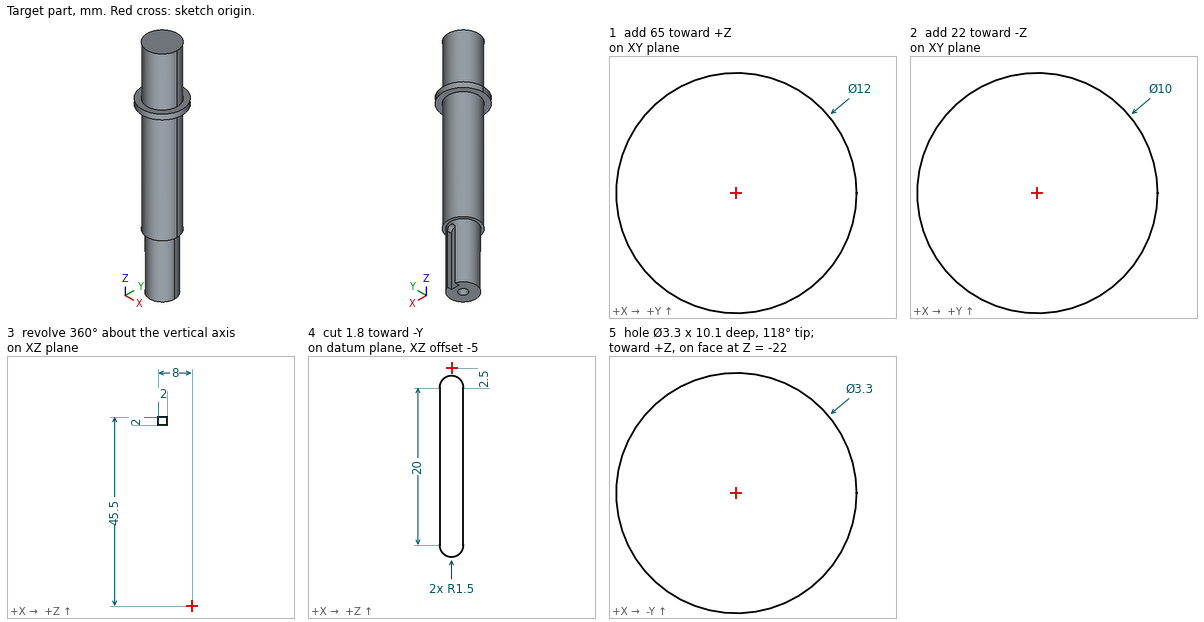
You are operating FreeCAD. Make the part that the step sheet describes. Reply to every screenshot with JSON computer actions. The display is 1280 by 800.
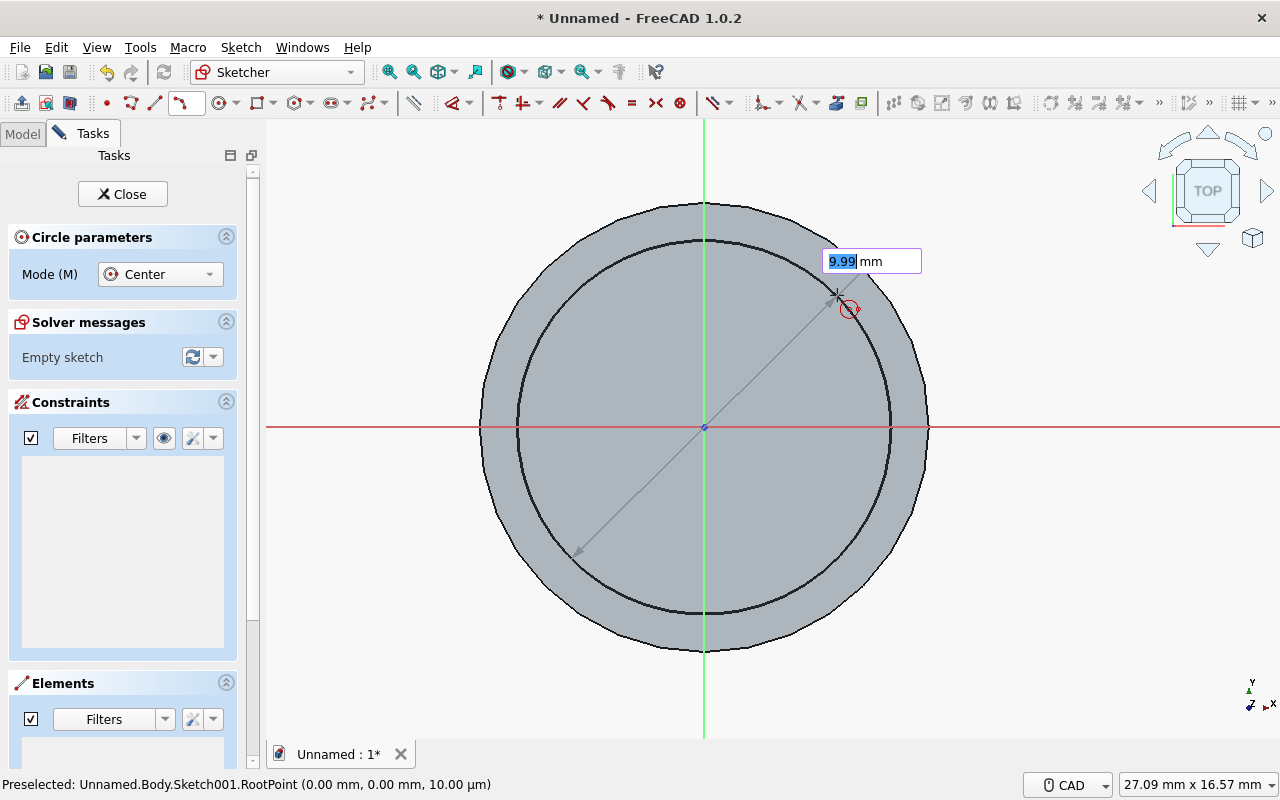
{"action": "type", "text": "10"}
{"action": "key", "text": "Return"}
{"action": "key", "text": "Escape"}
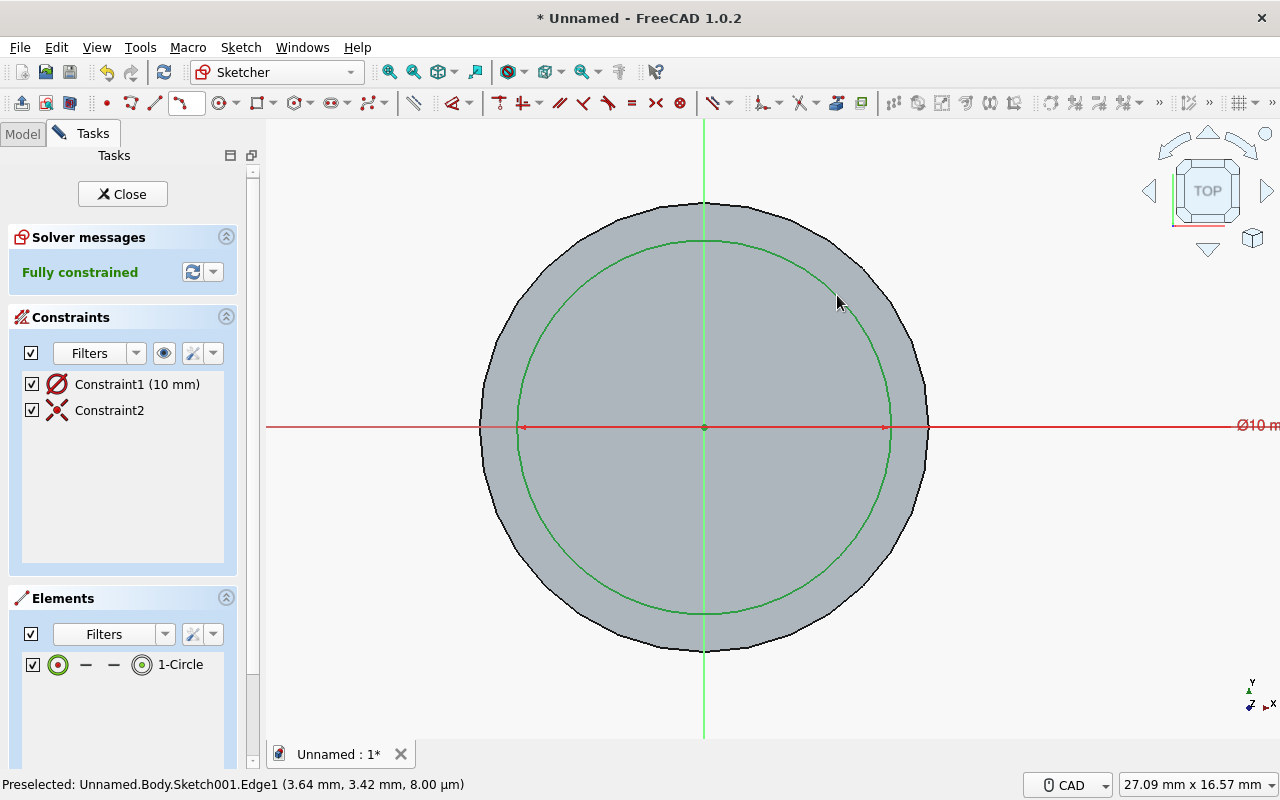
{"action": "left_click", "coordinate": [123, 194]}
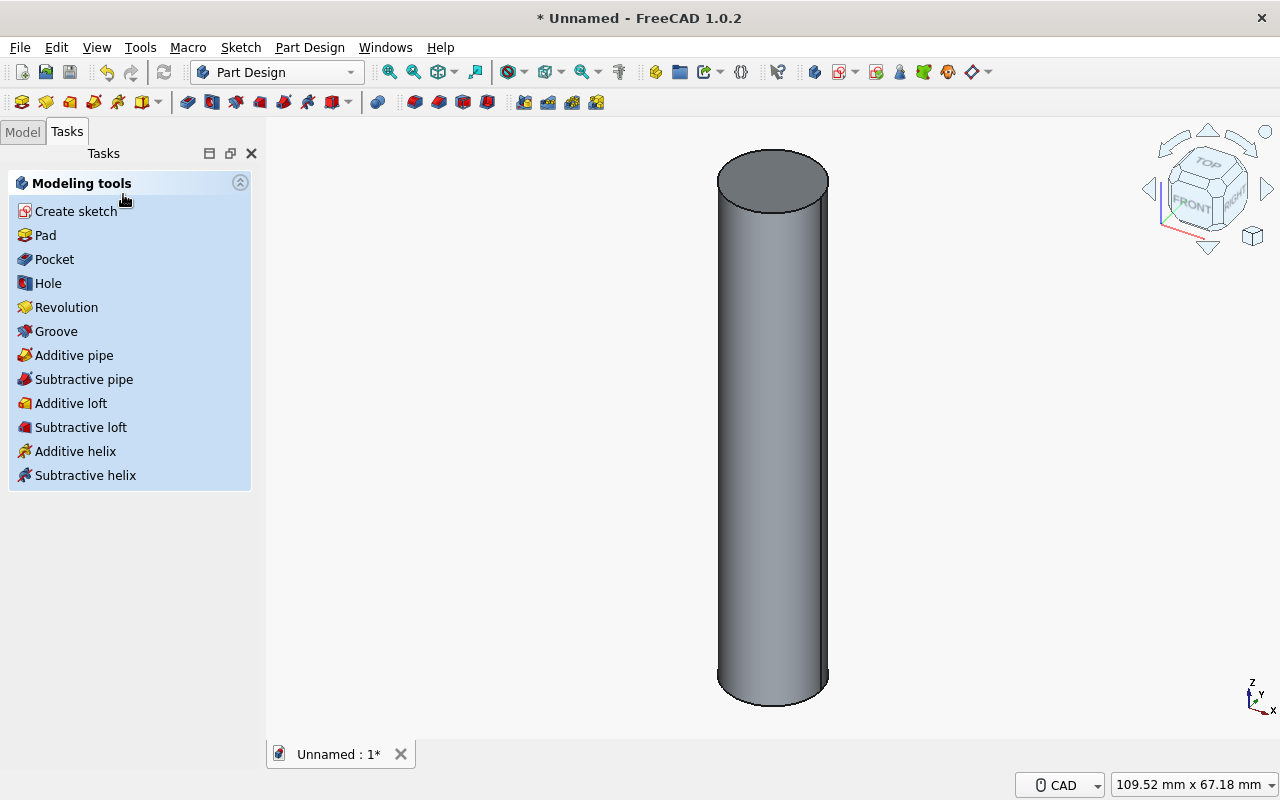
{"action": "left_click", "coordinate": [22, 102]}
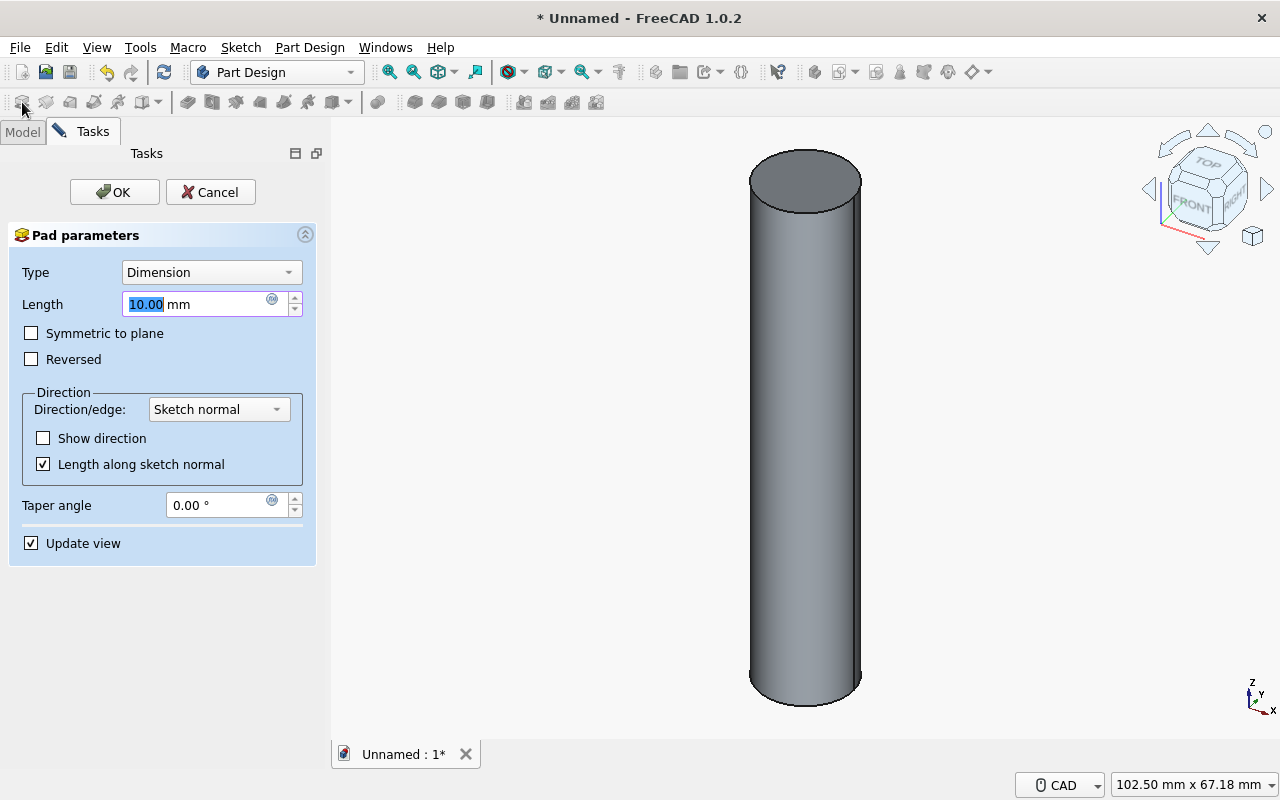
{"action": "type", "text": "22"}
{"action": "key", "text": "Tab"}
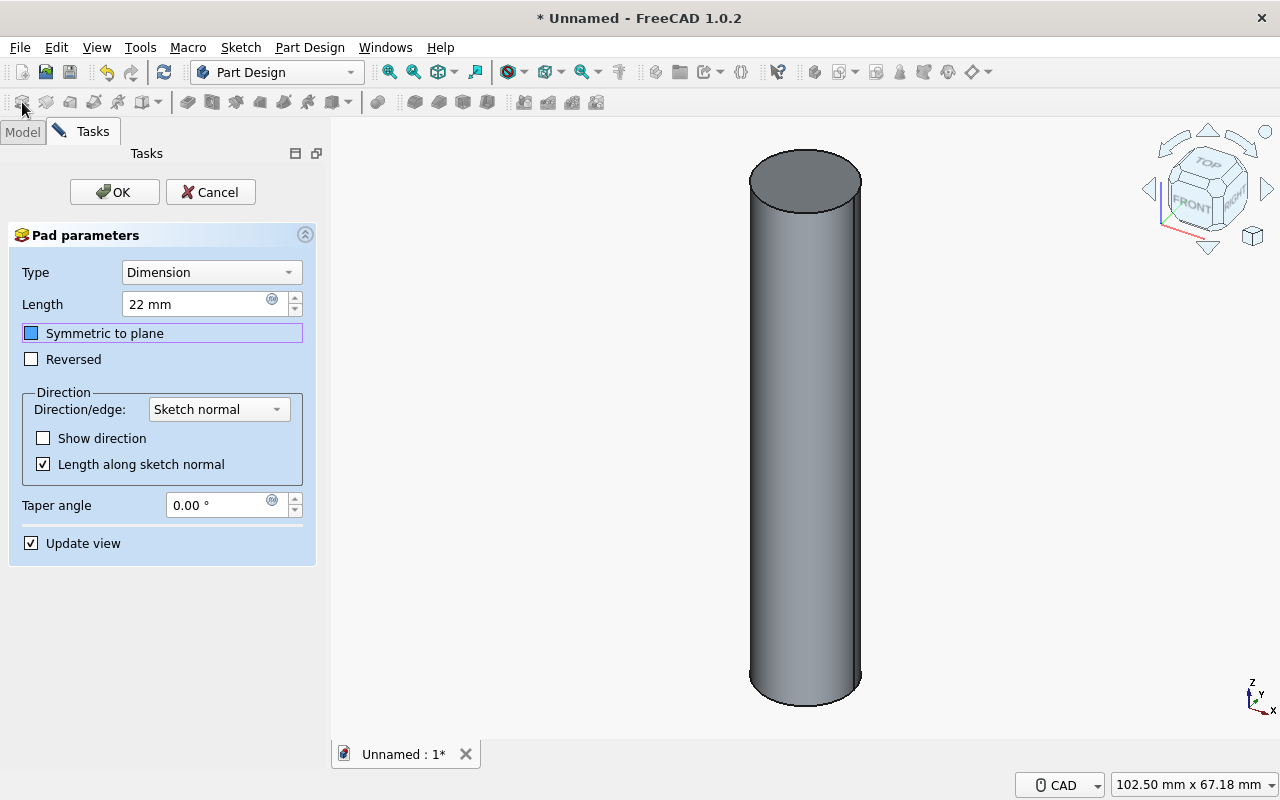
{"action": "left_click", "coordinate": [30, 359]}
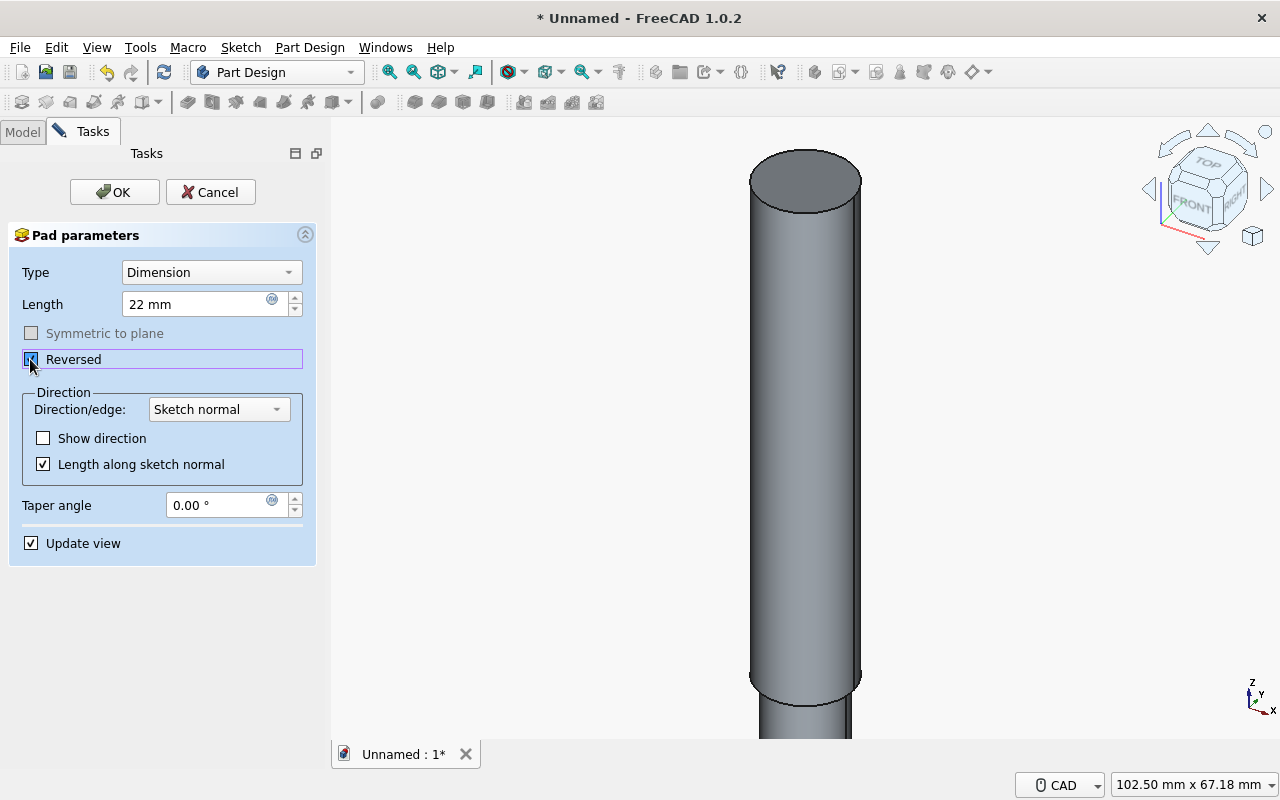
{"action": "left_click", "coordinate": [115, 192]}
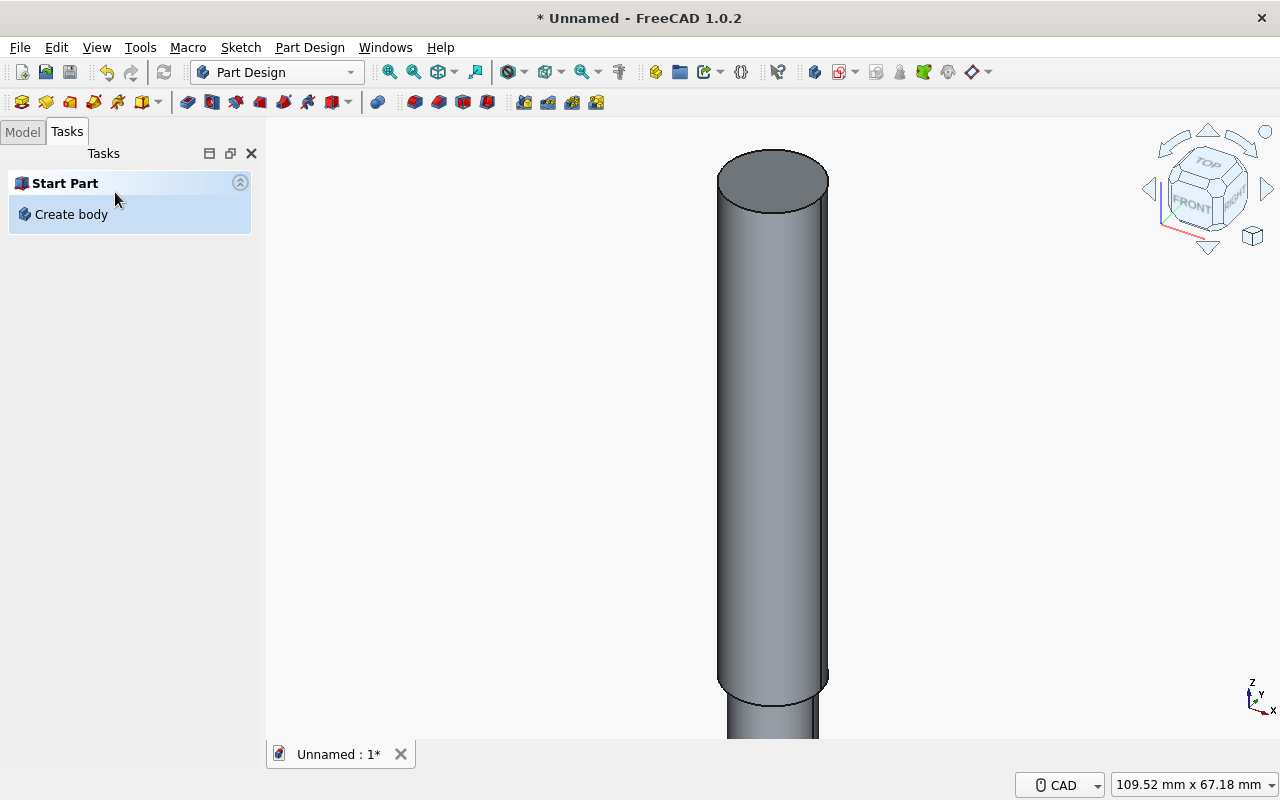
{"action": "left_click", "coordinate": [390, 72]}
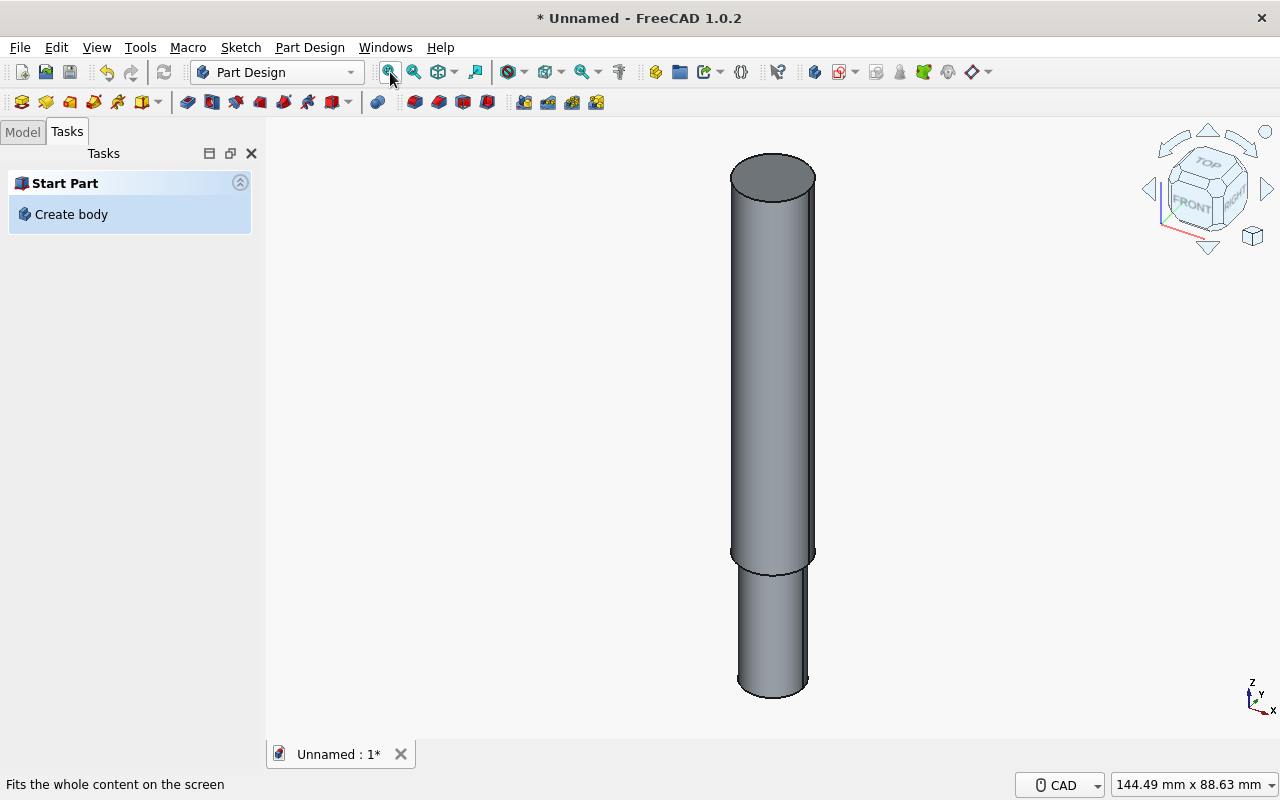
{"action": "left_click", "coordinate": [840, 72]}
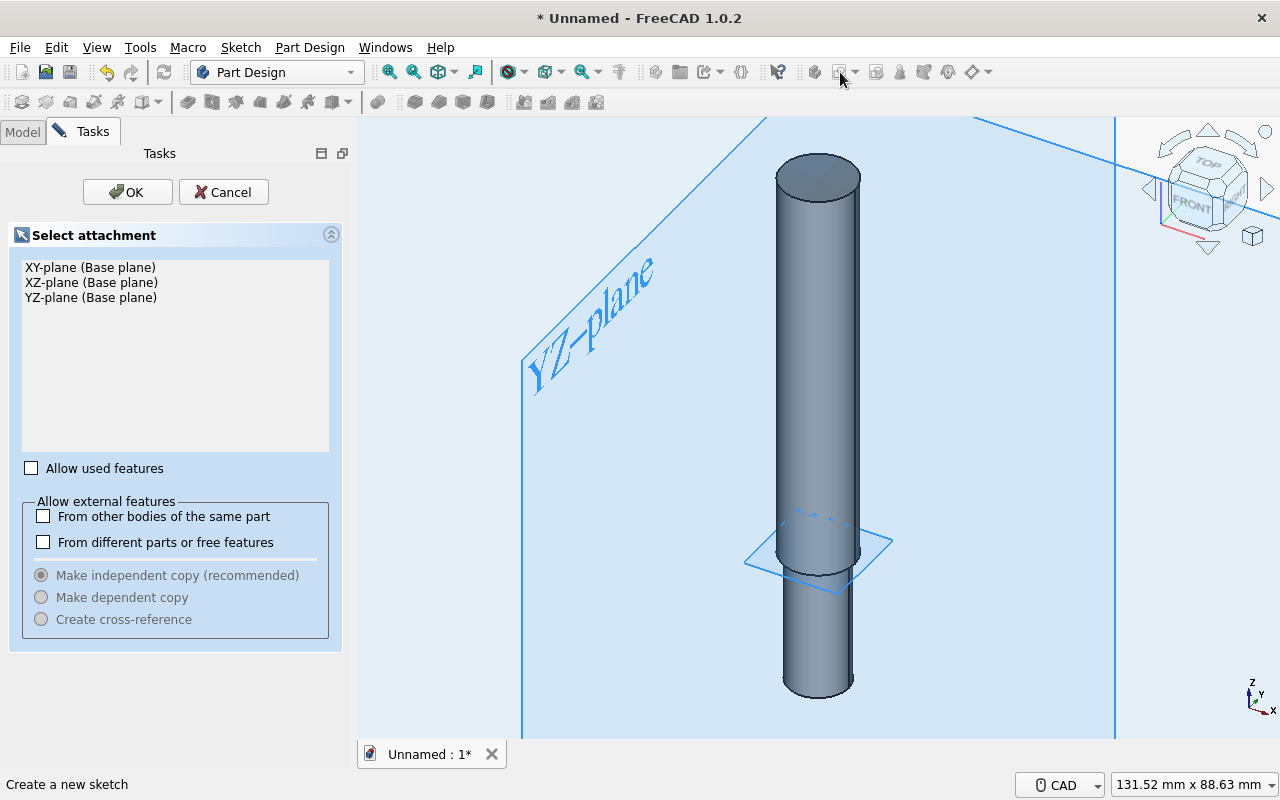
{"action": "left_click", "coordinate": [82, 282]}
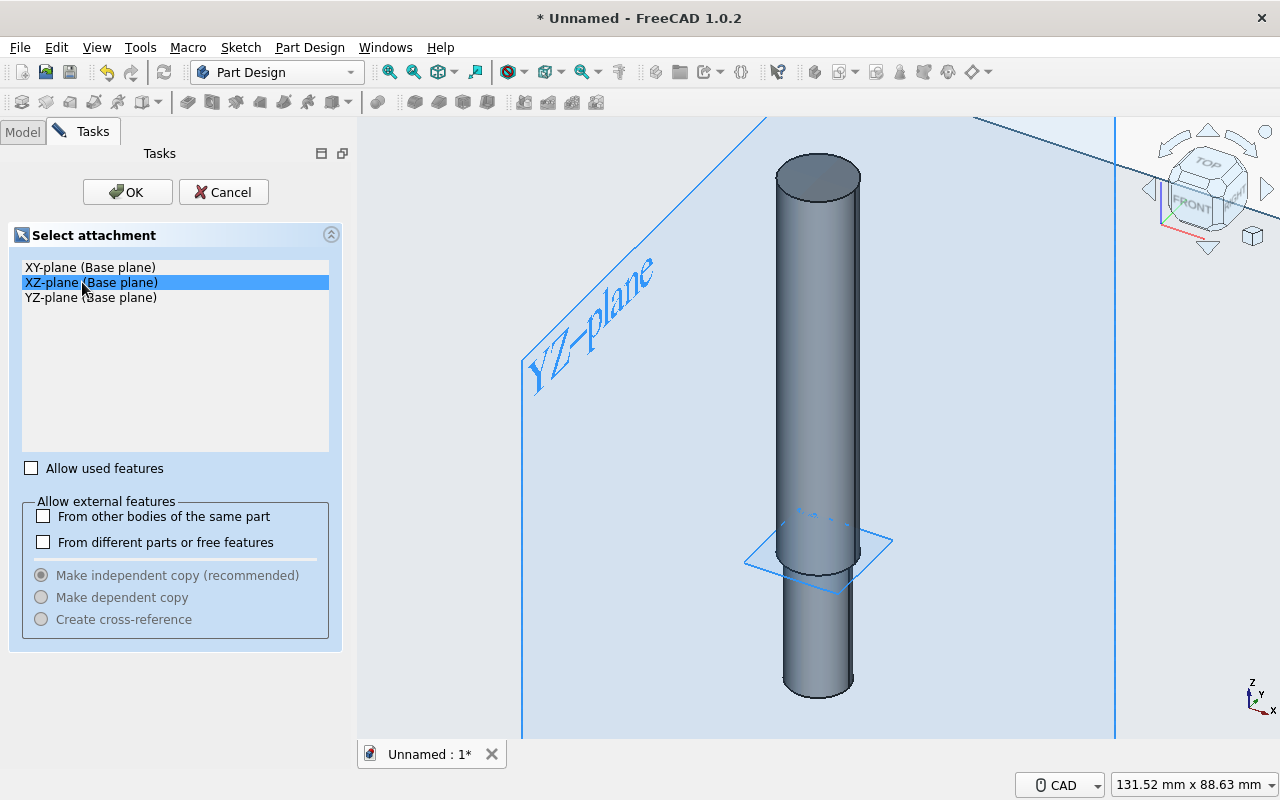
{"action": "left_click", "coordinate": [128, 192]}